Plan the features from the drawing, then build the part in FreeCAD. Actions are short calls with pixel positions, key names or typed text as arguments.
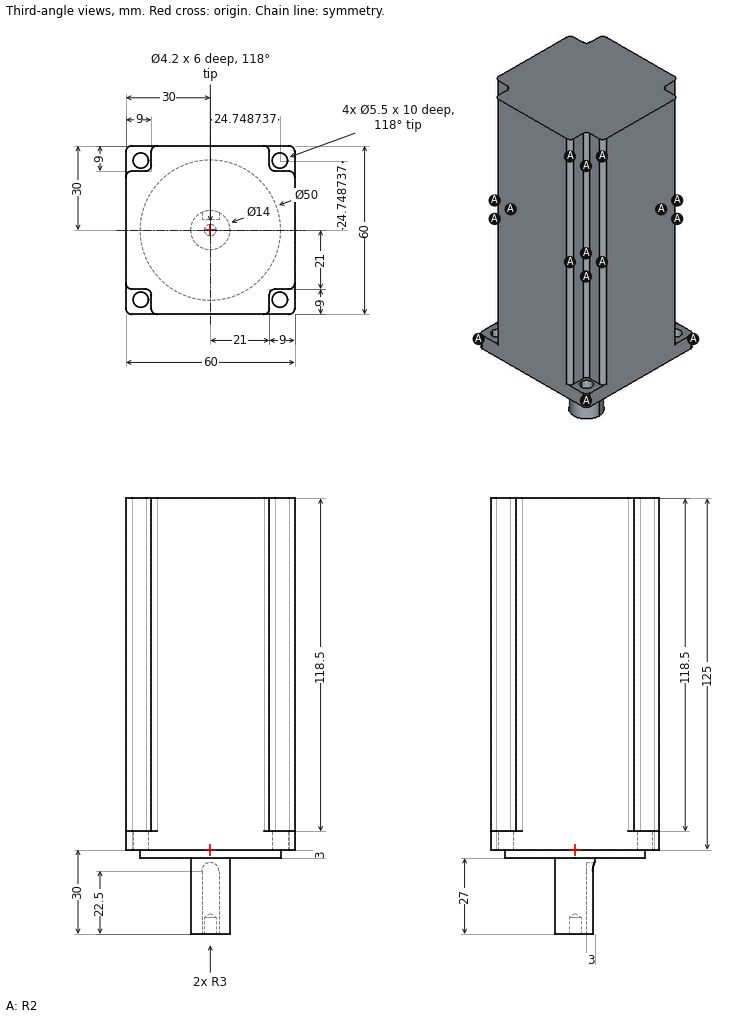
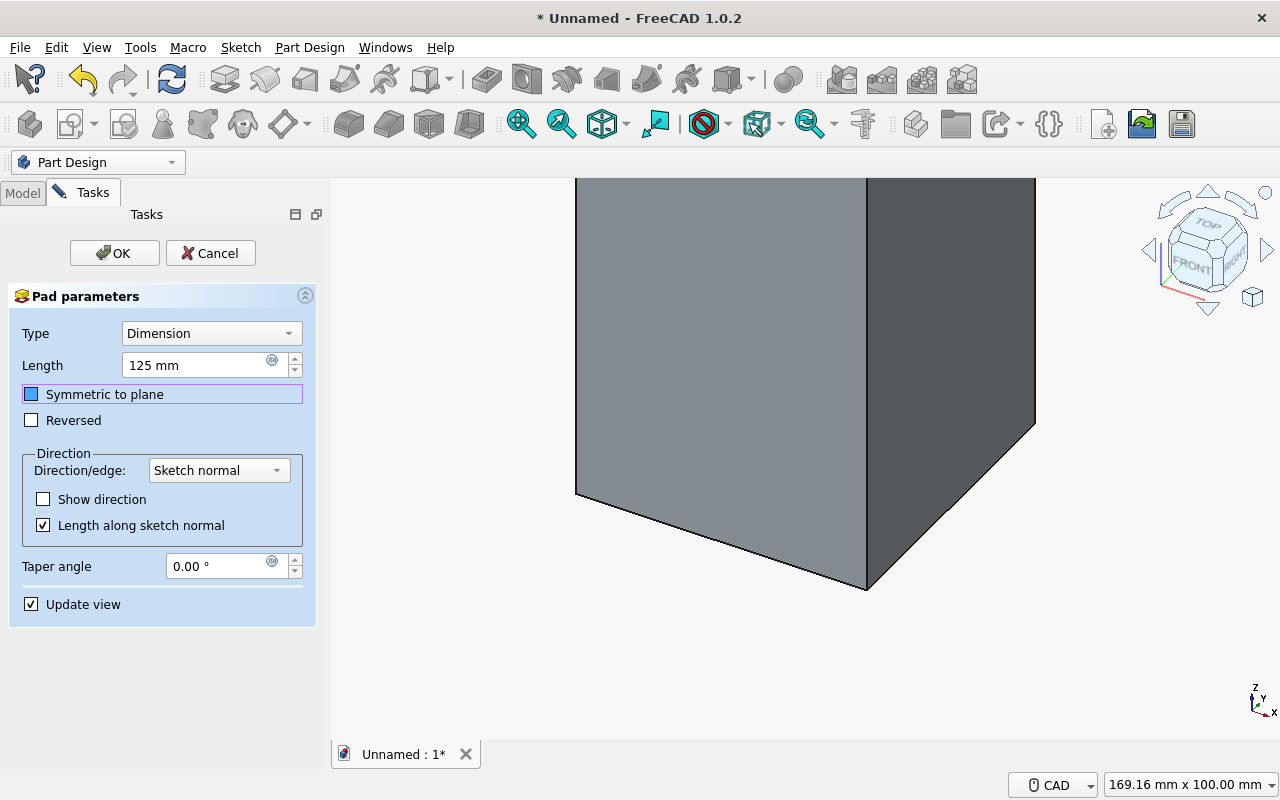
click(115, 253)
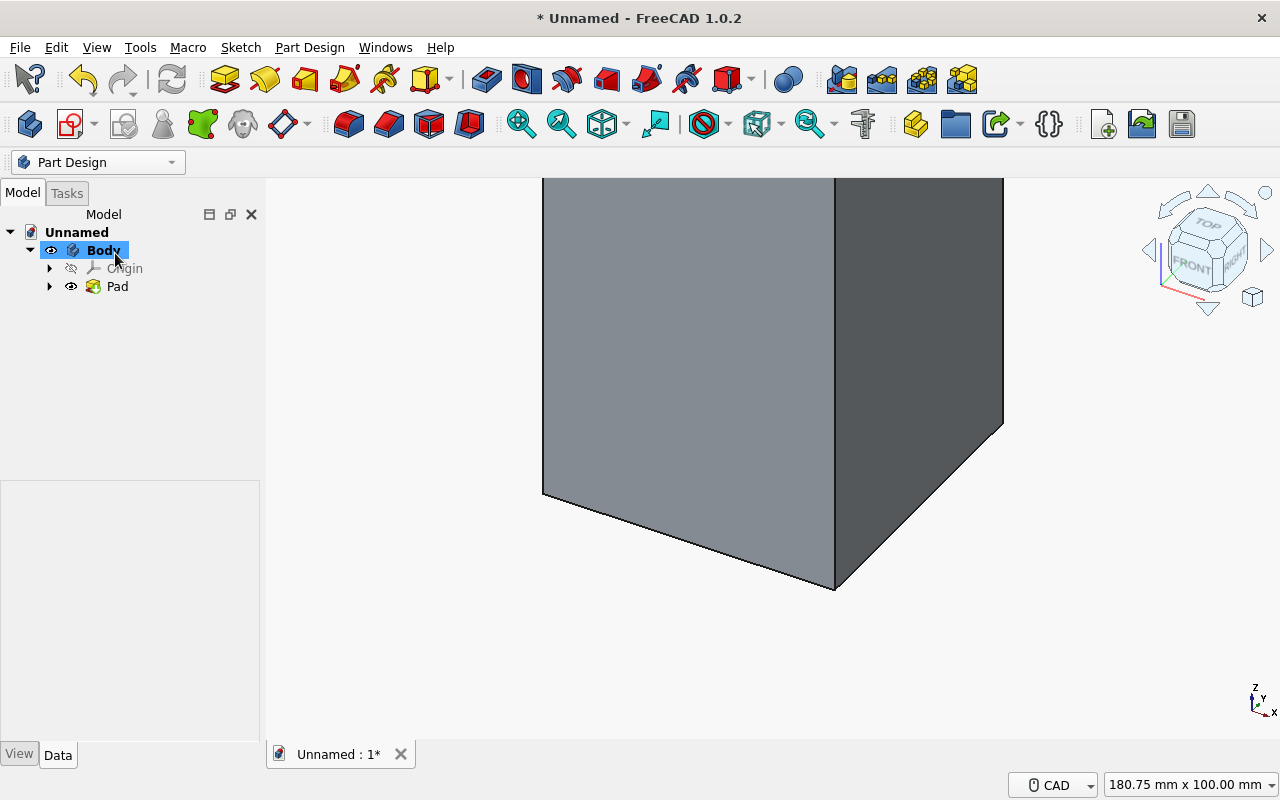
click(522, 124)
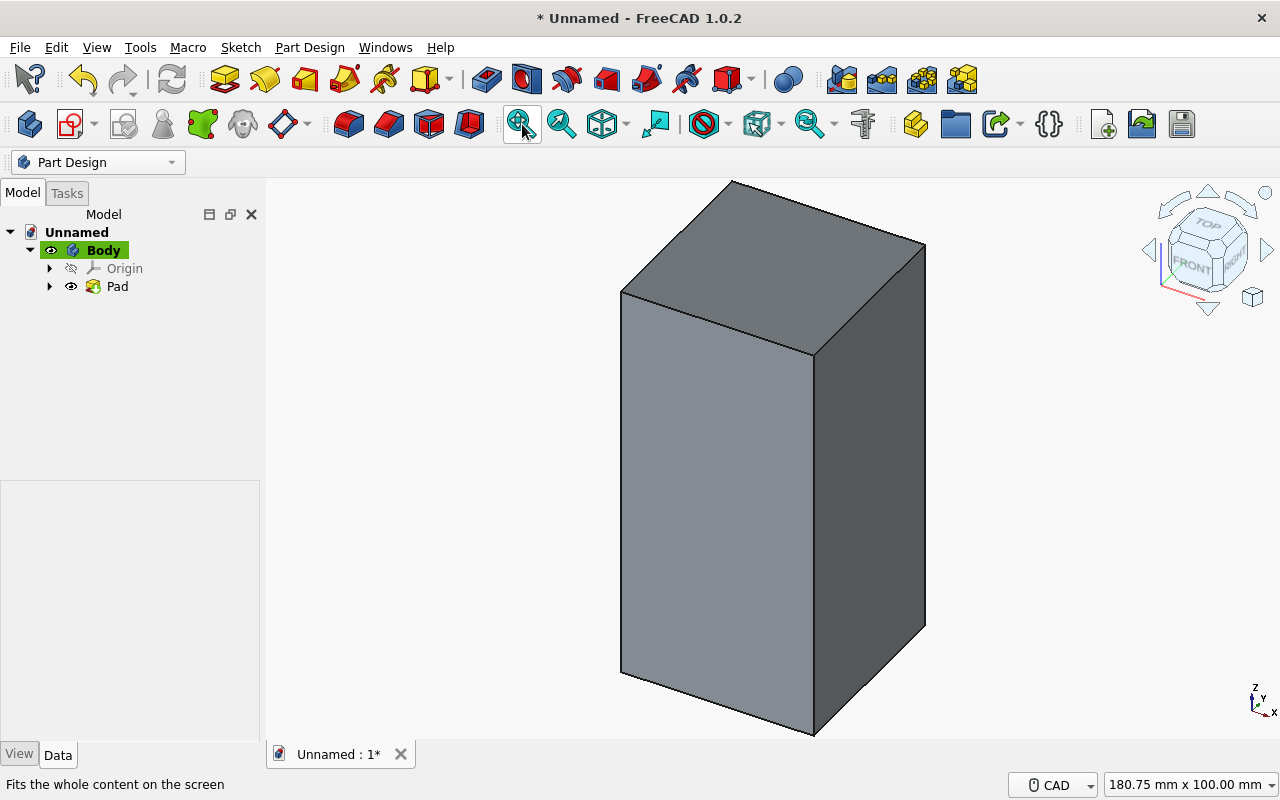
click(70, 124)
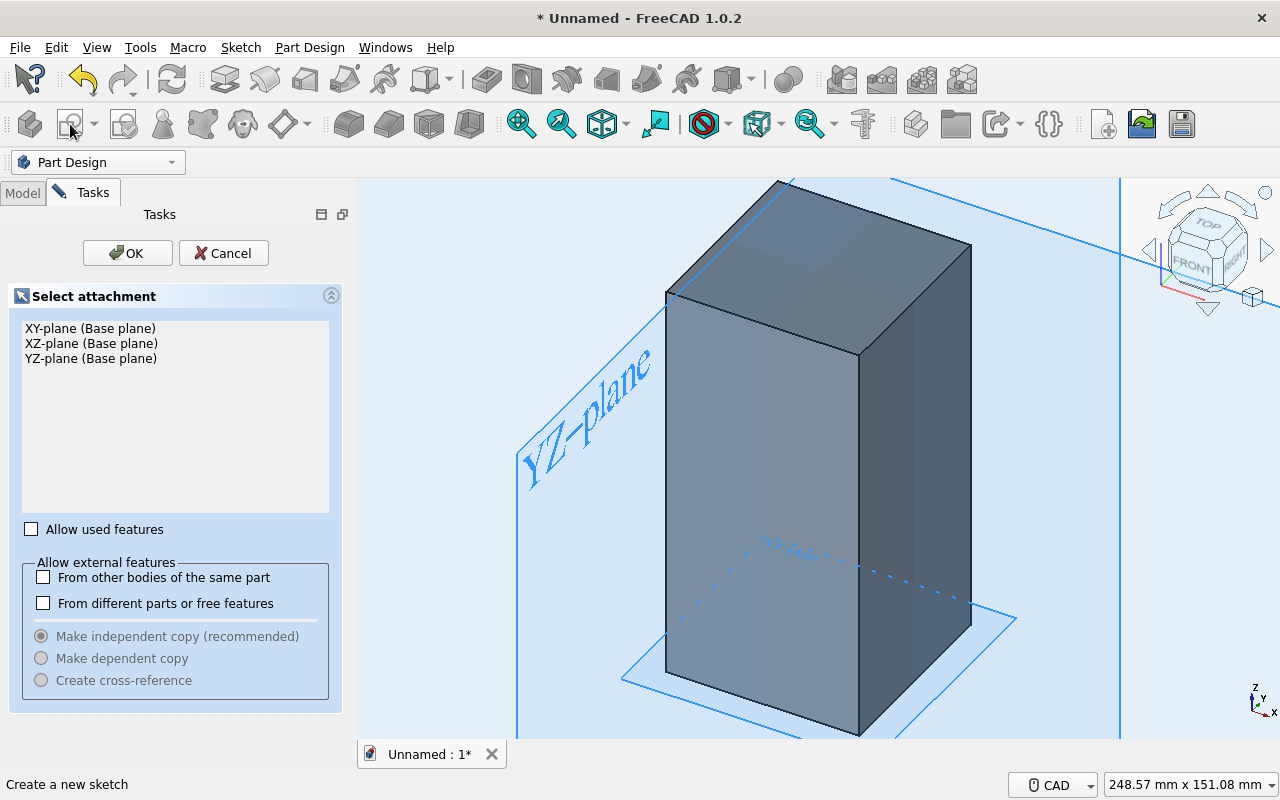
click(82, 328)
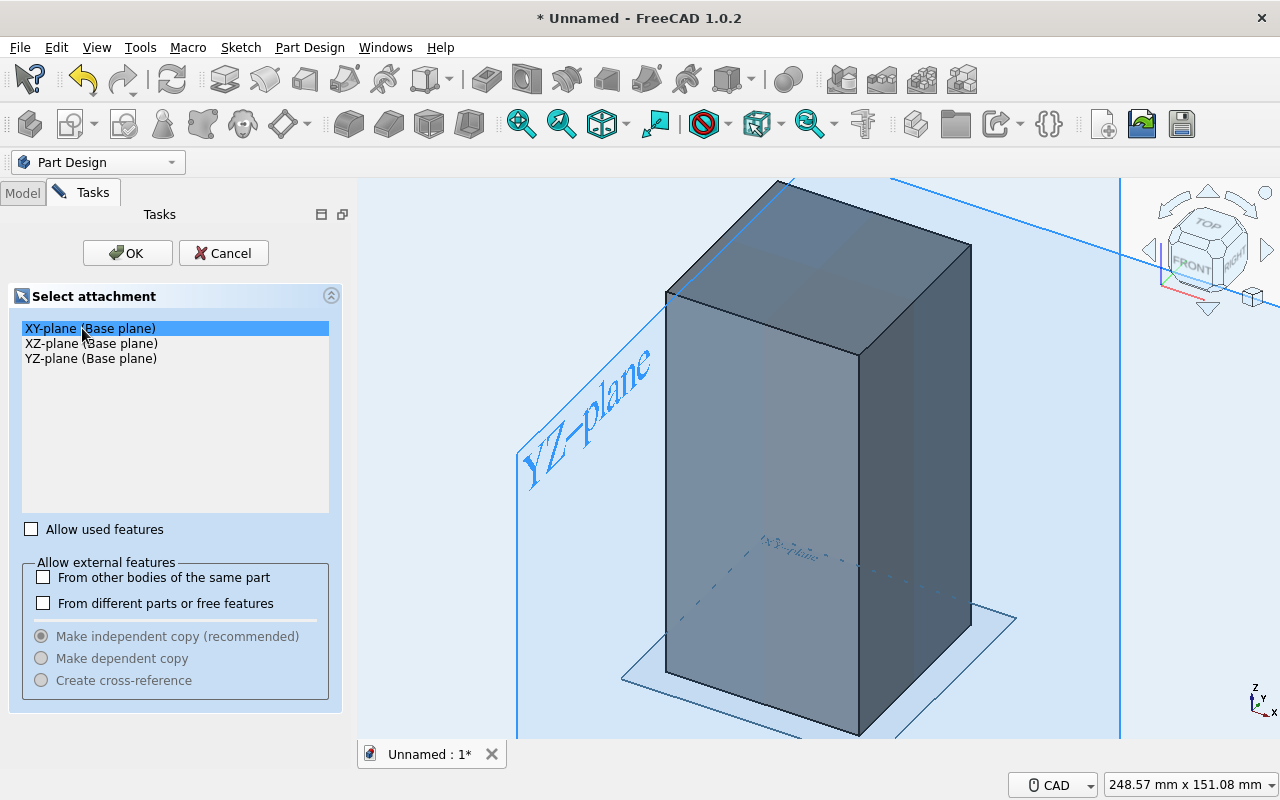
click(128, 253)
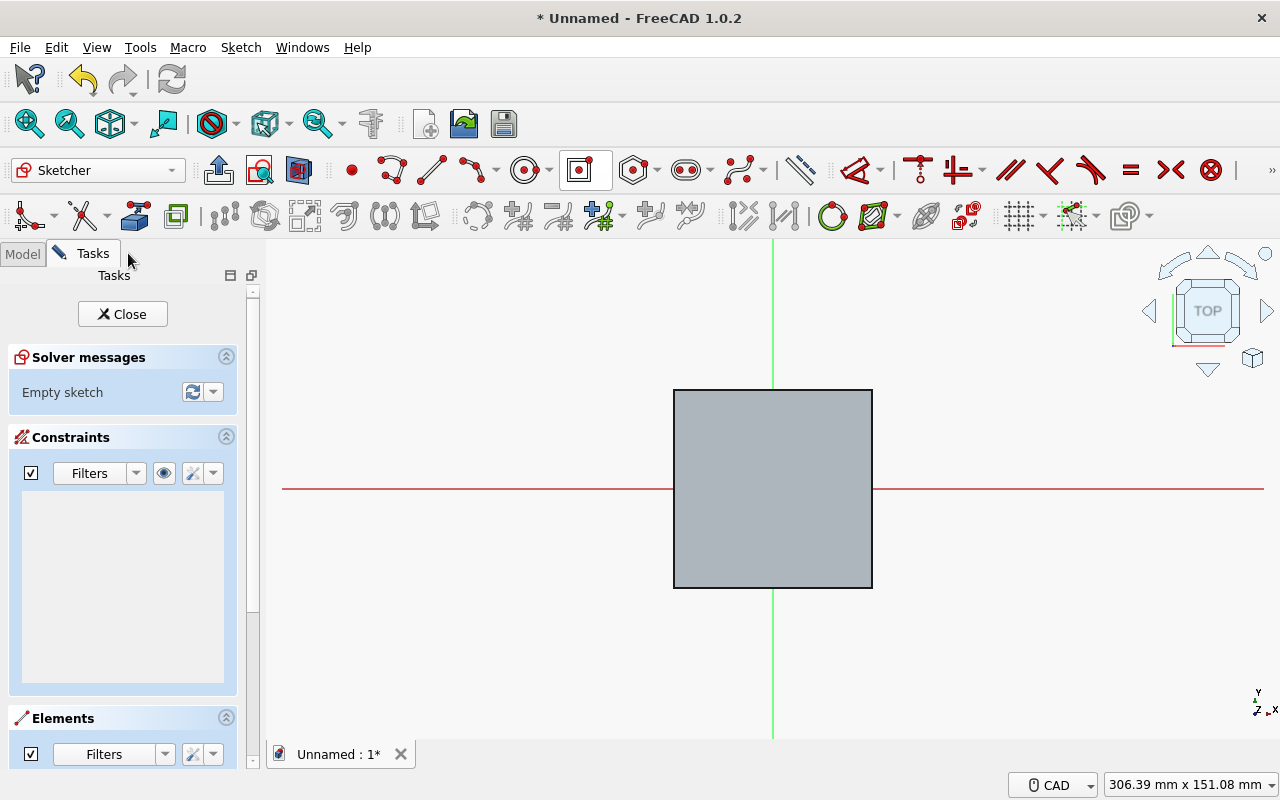
click(300, 170)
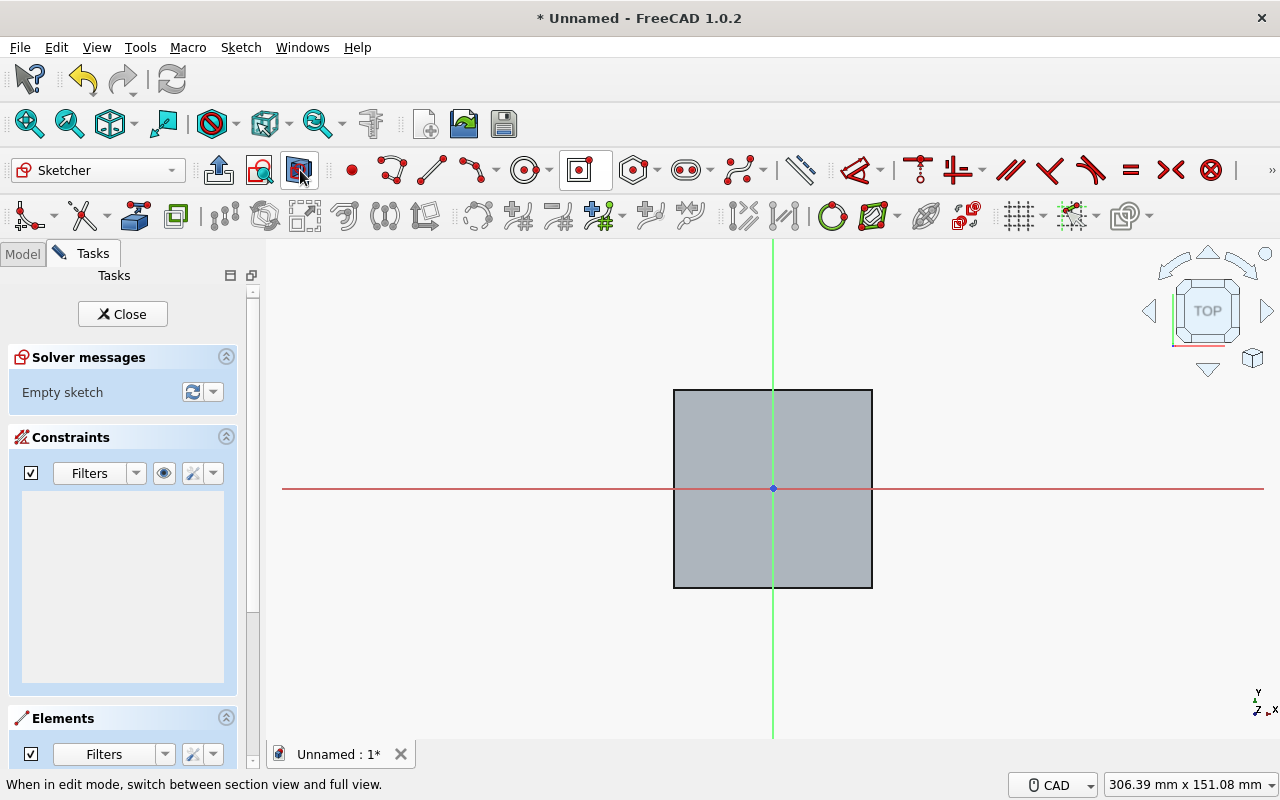
scroll(856, 489, up, 3)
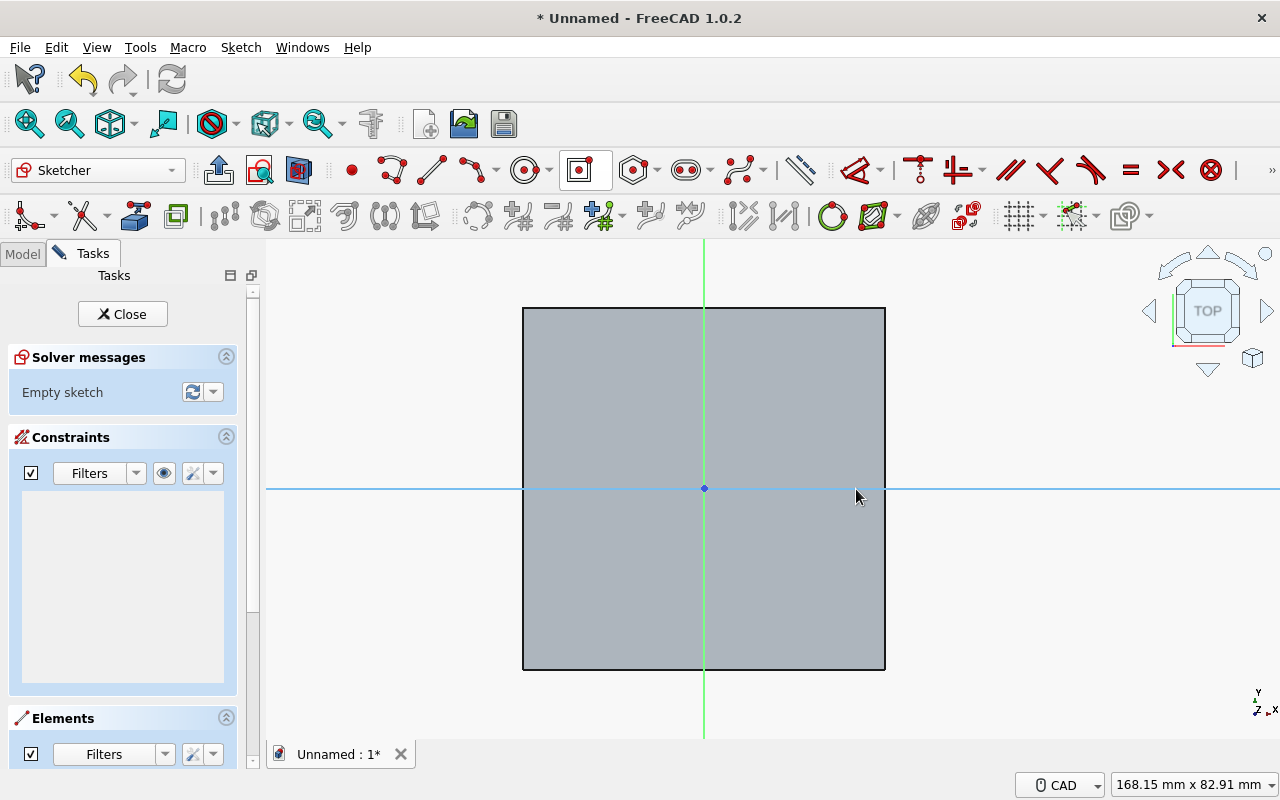
click(526, 170)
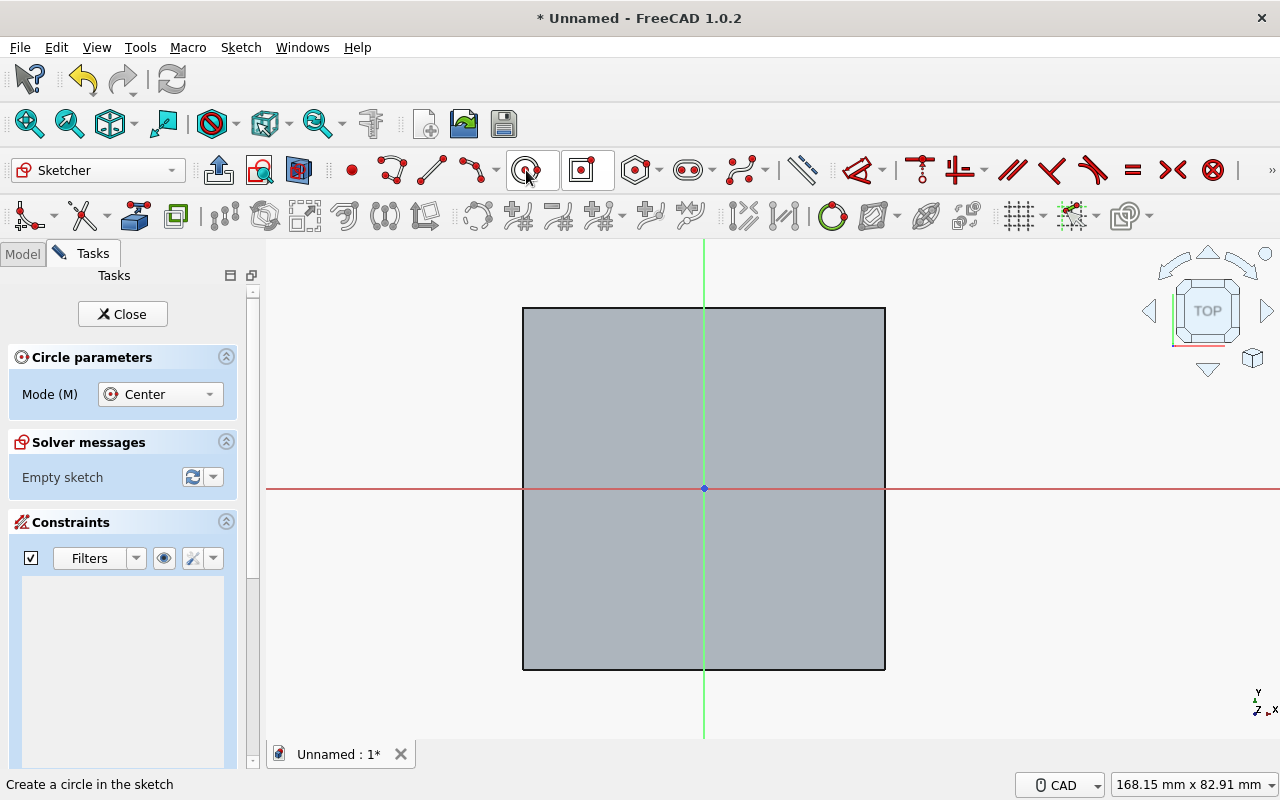
click(704, 489)
move(811, 382)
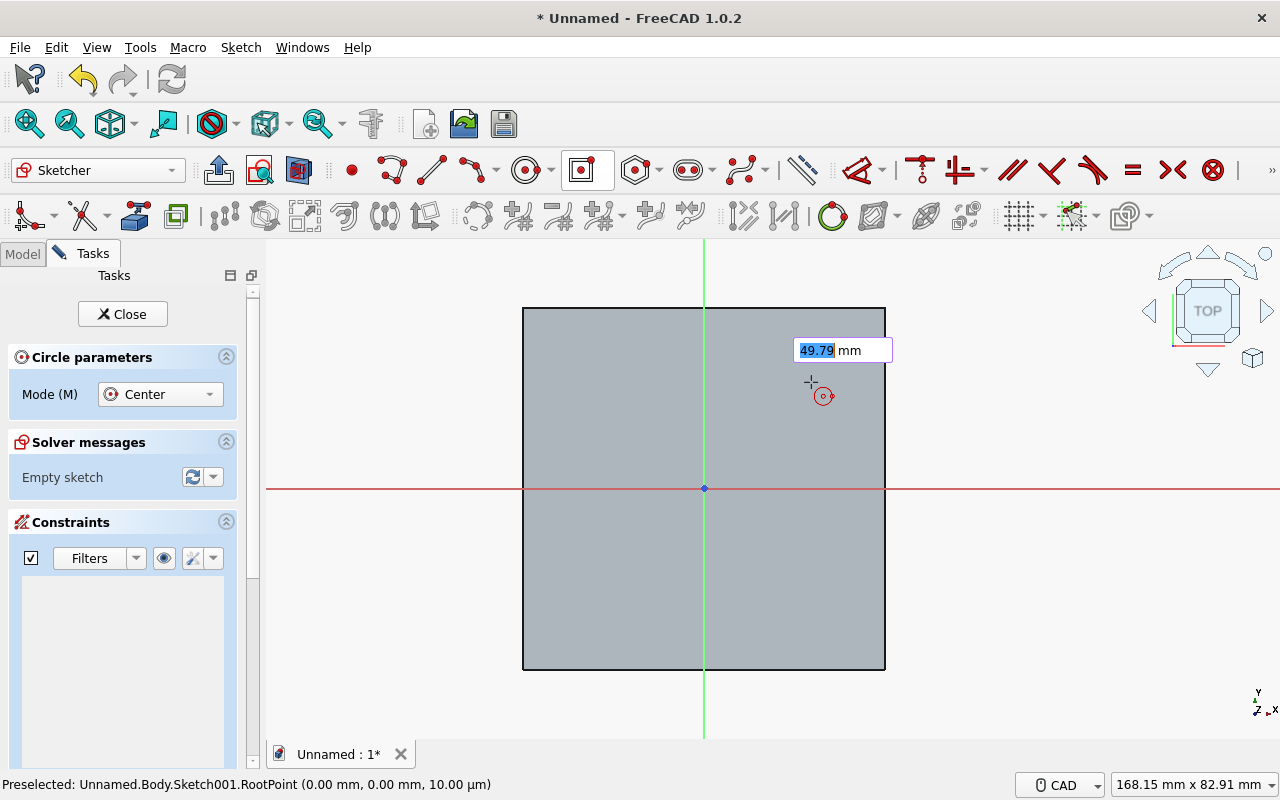
text(50)
key(Return)
key(Escape)